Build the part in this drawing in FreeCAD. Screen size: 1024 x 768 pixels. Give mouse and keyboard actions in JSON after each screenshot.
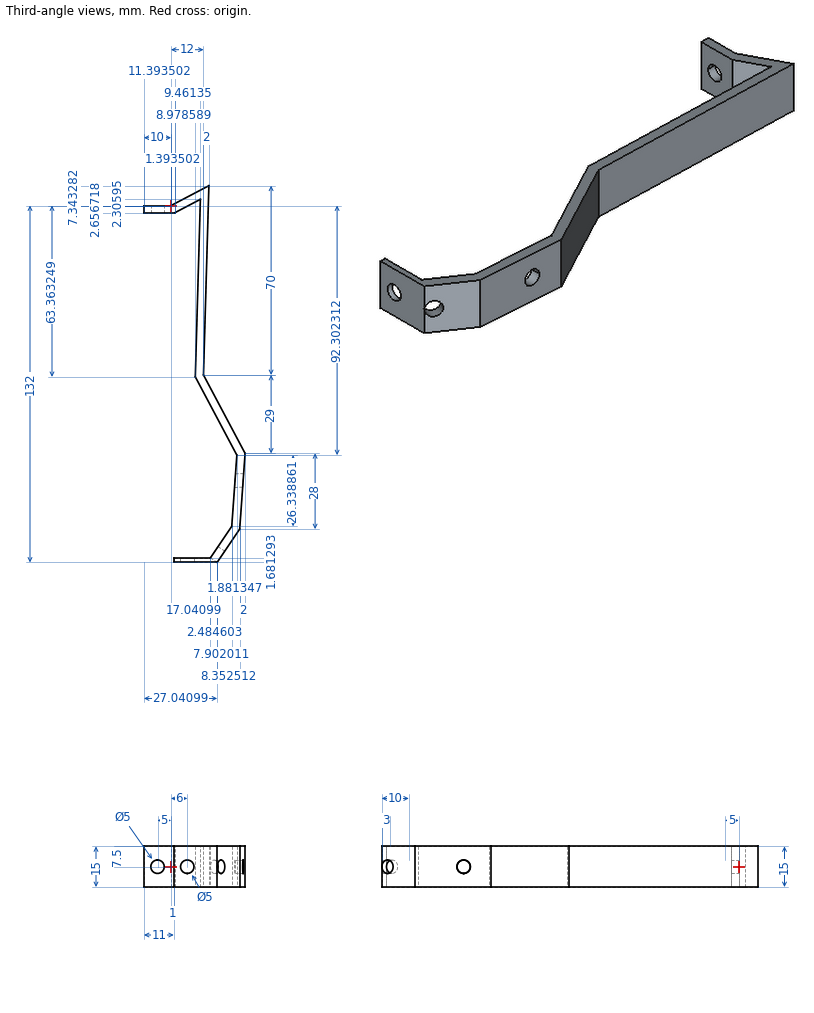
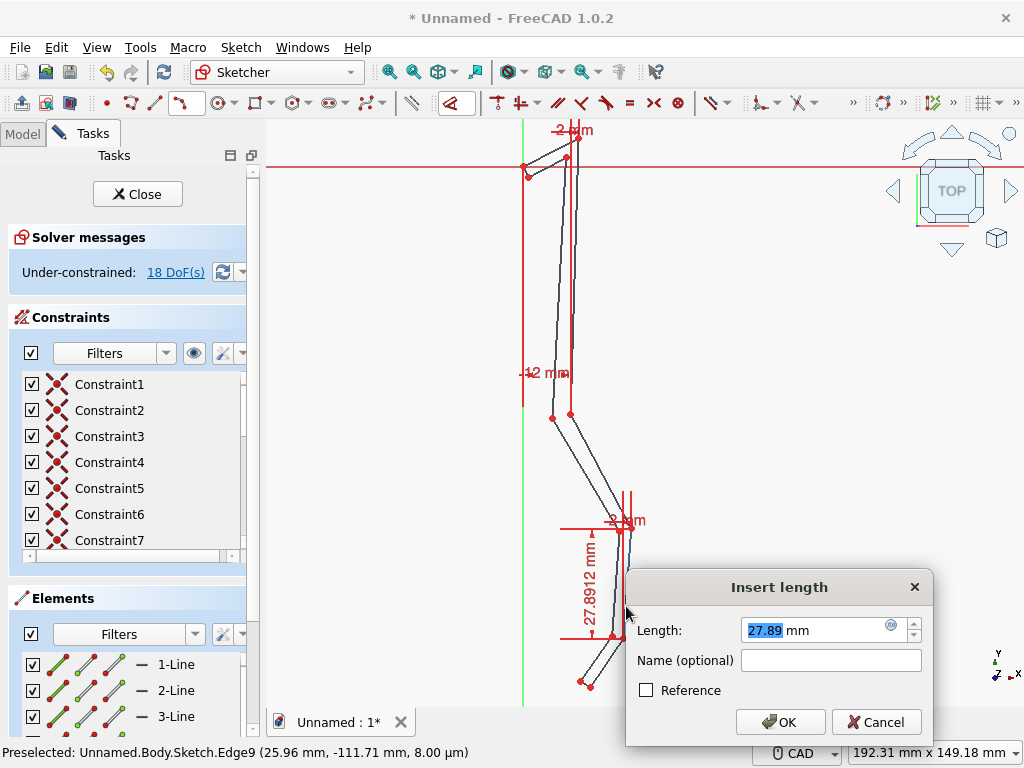
{"action": "type", "text": "28"}
{"action": "key", "text": "Return"}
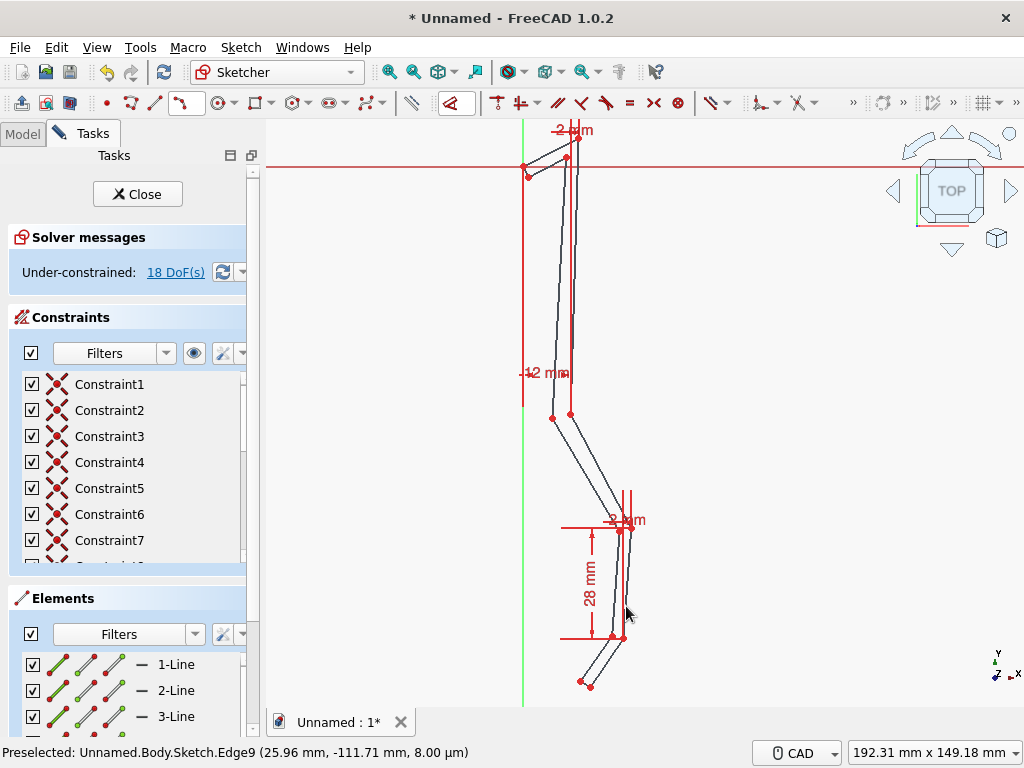
{"action": "left_click", "coordinate": [613, 494]}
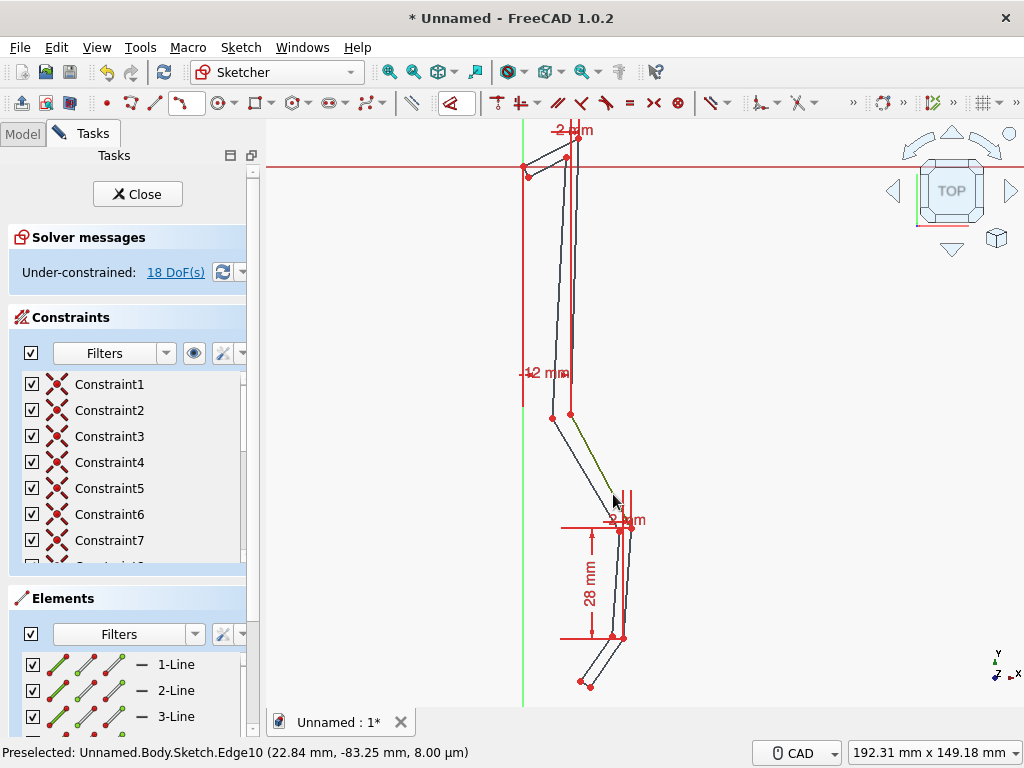
{"action": "key", "text": "i"}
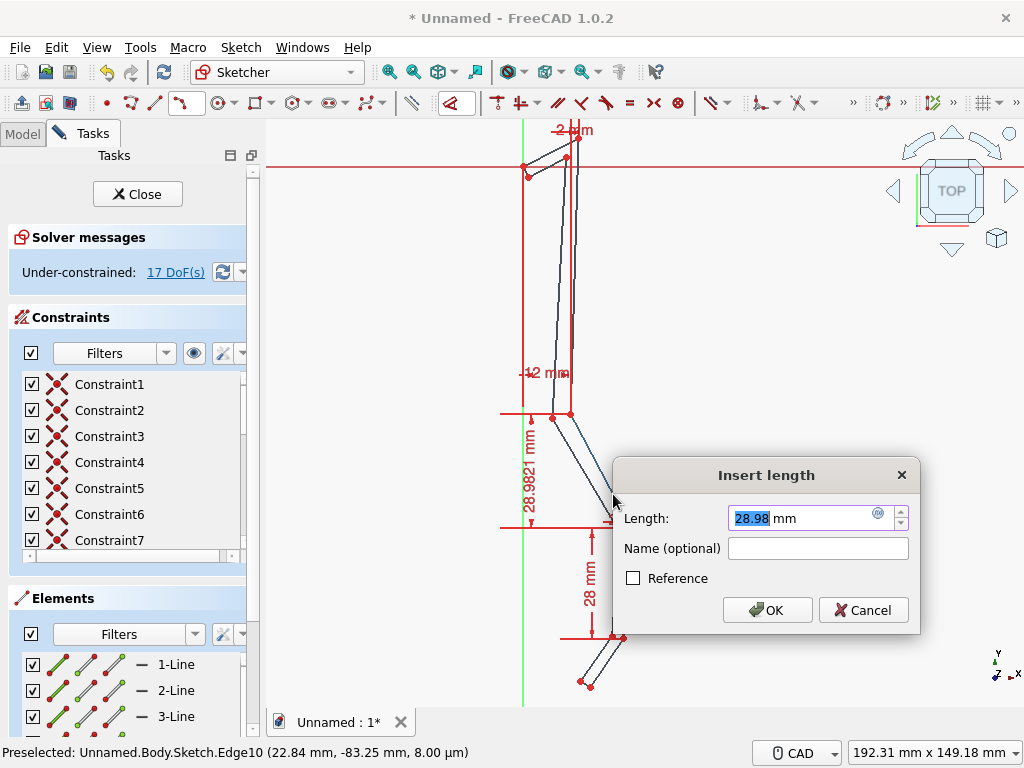
{"action": "type", "text": "29"}
{"action": "key", "text": "Return"}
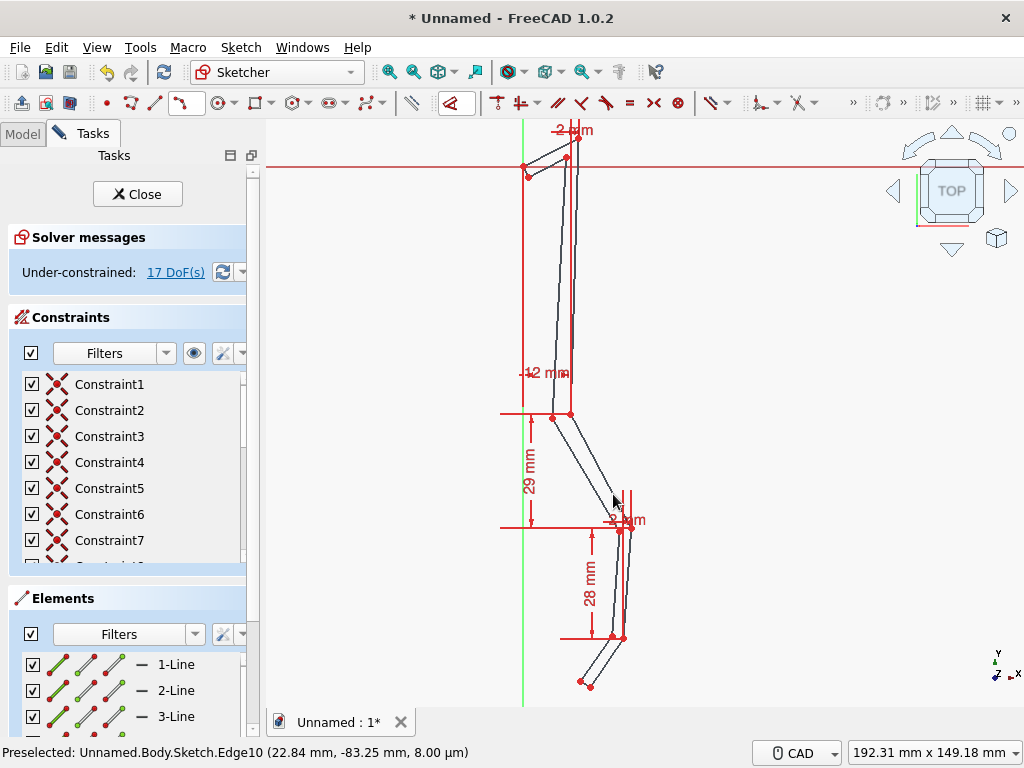
{"action": "left_click", "coordinate": [573, 332]}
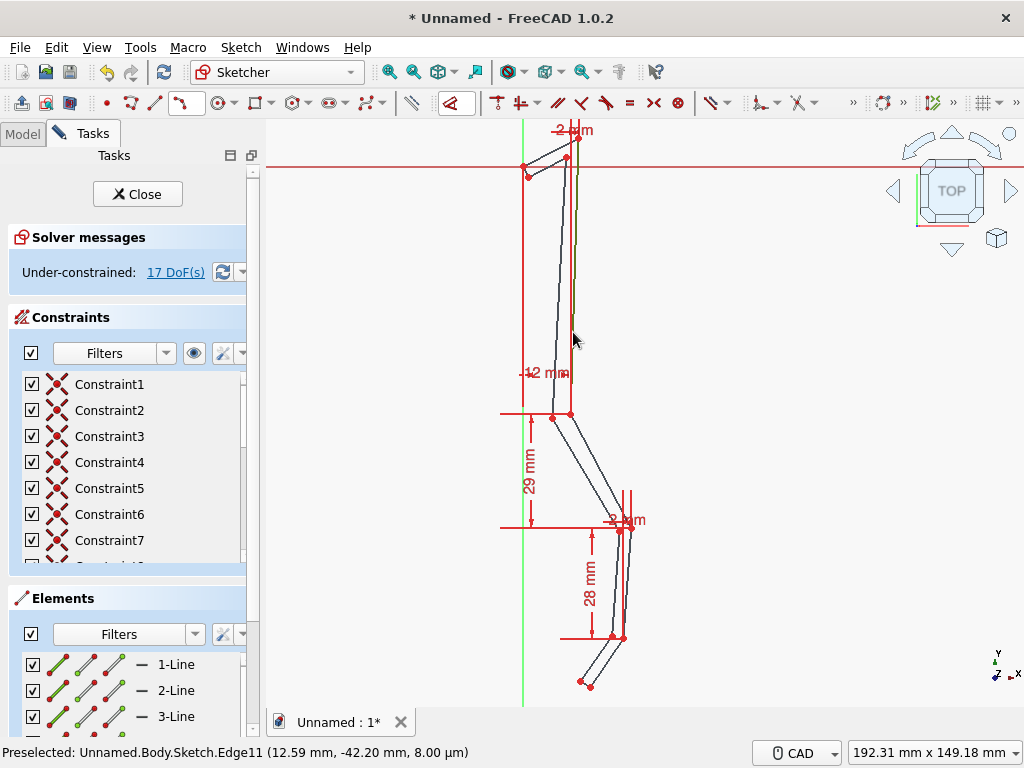
{"action": "left_click", "coordinate": [470, 104]}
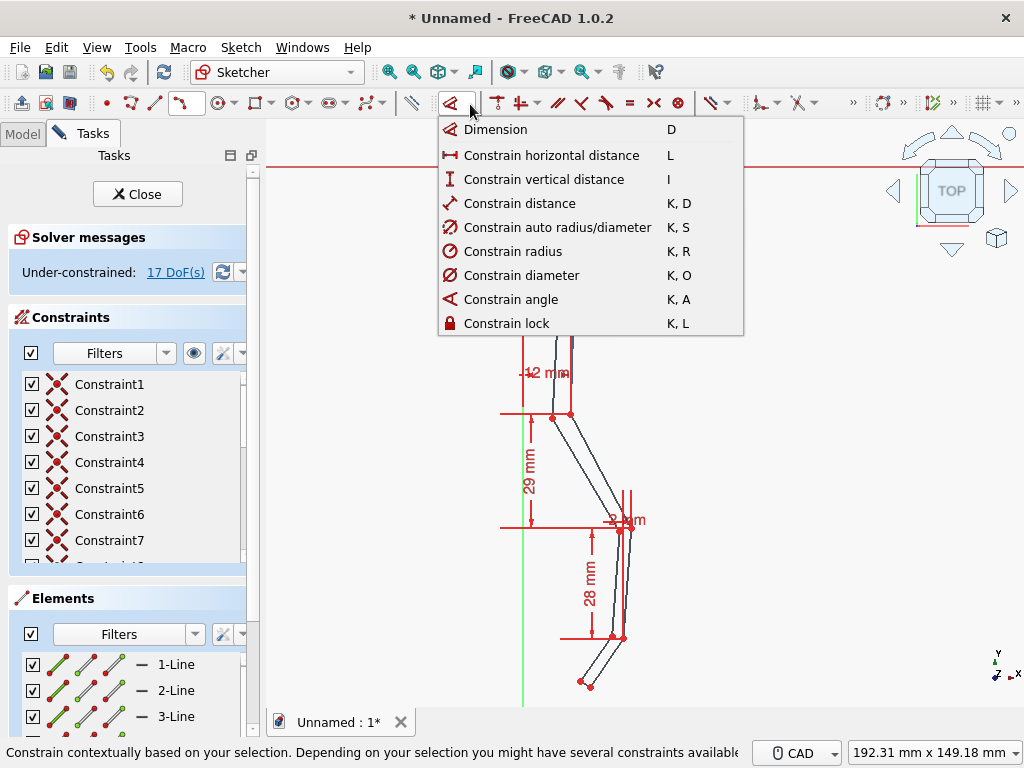
{"action": "left_click", "coordinate": [591, 179]}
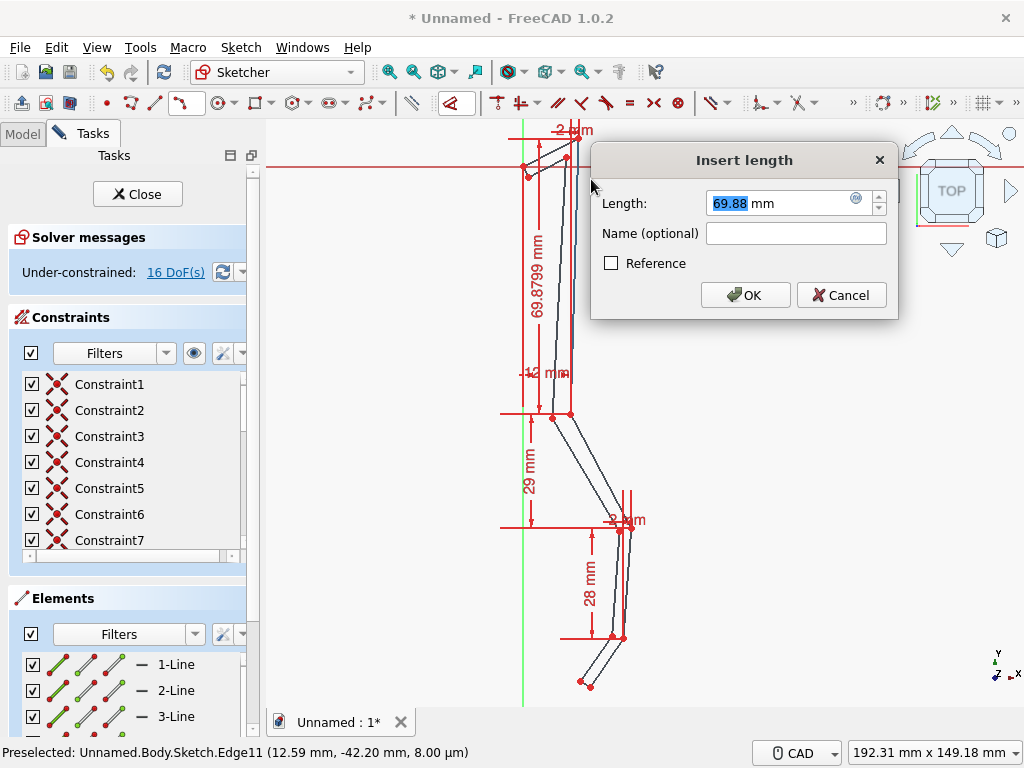
{"action": "type", "text": "70"}
{"action": "key", "text": "Return"}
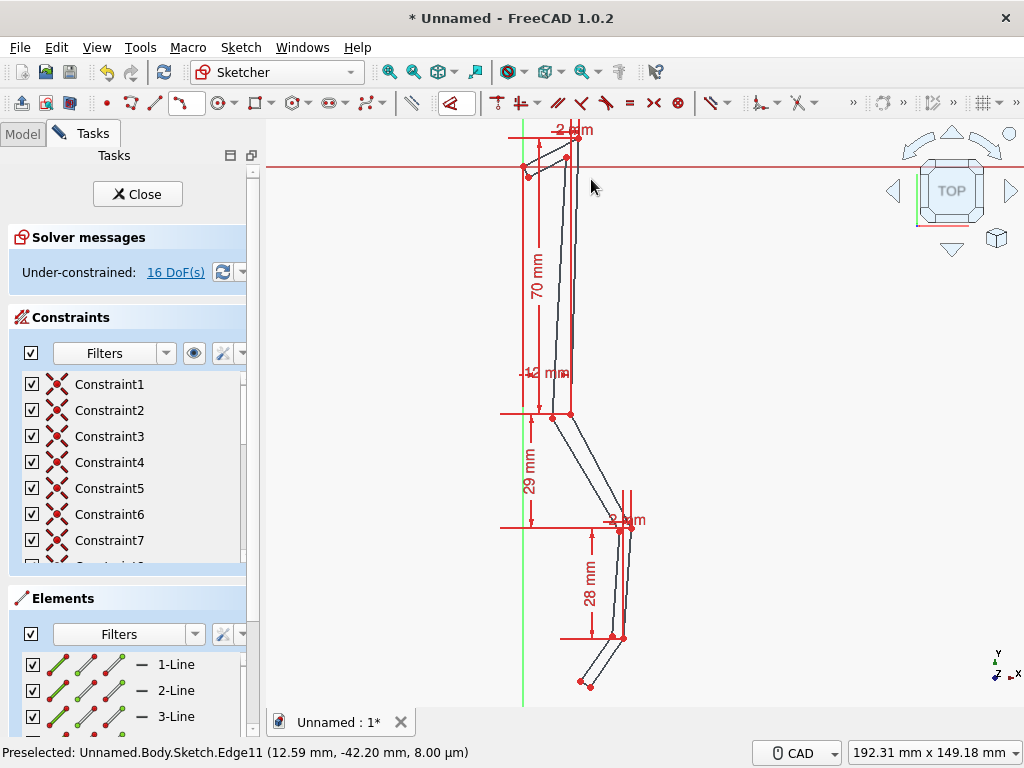
{"action": "scroll", "coordinate": [575, 414], "scroll_direction": "down", "scroll_amount": 2}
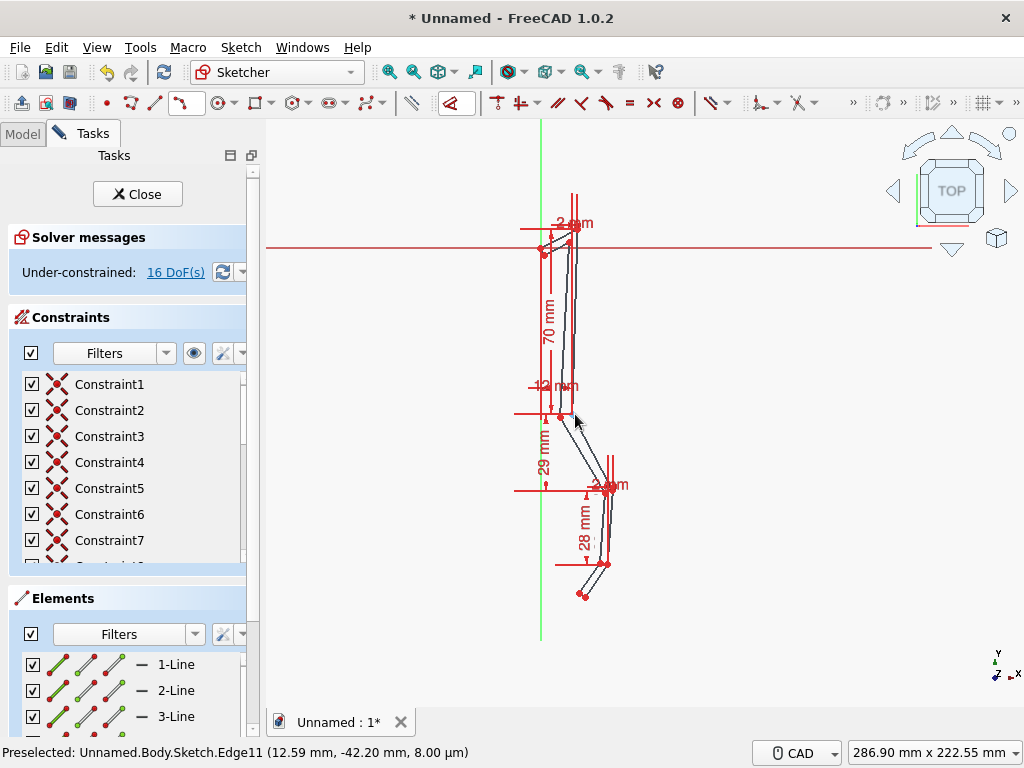
{"action": "scroll", "coordinate": [585, 598], "scroll_direction": "up", "scroll_amount": 3}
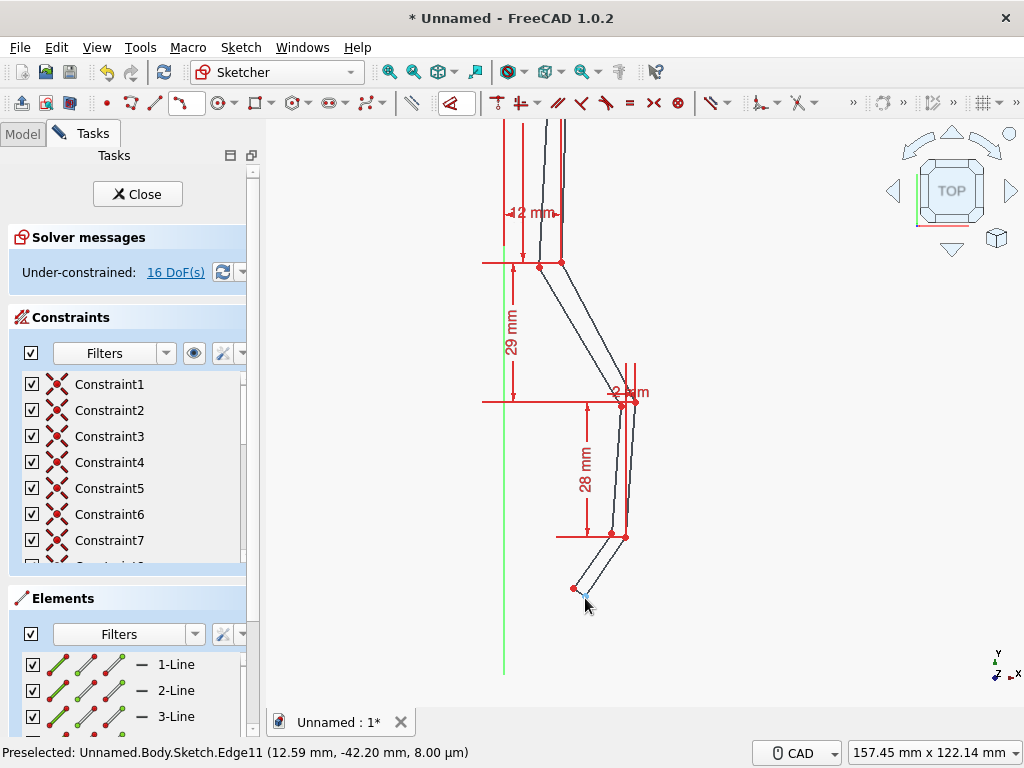
{"action": "left_click", "coordinate": [585, 597]}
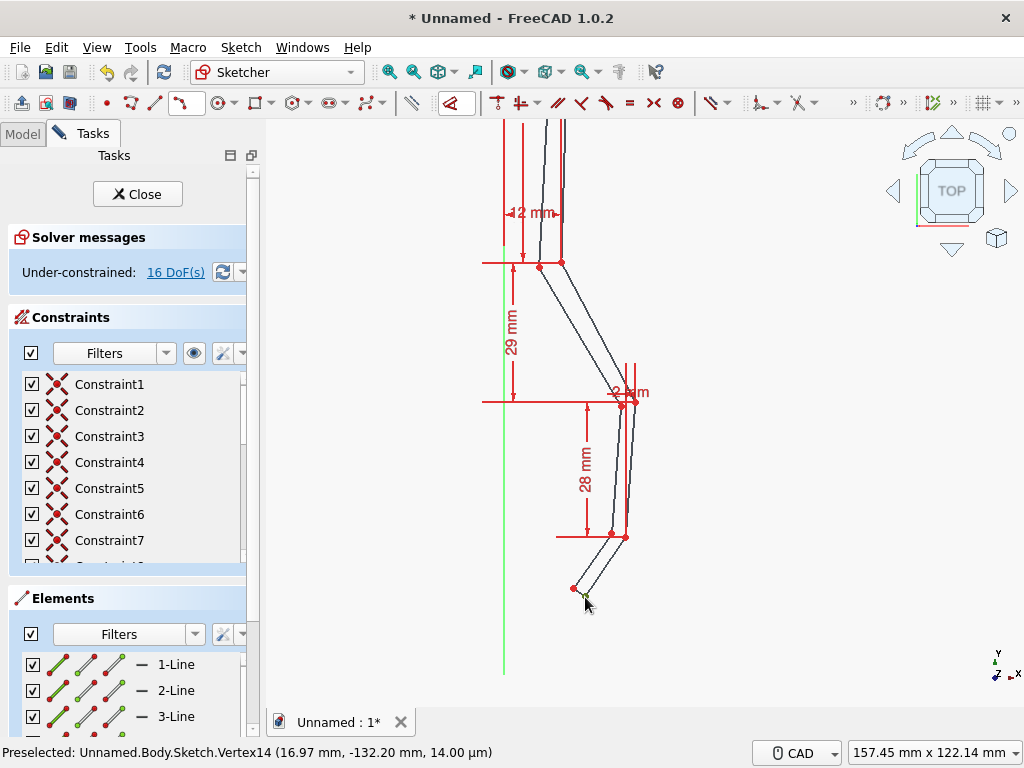
{"action": "left_click", "coordinate": [470, 104]}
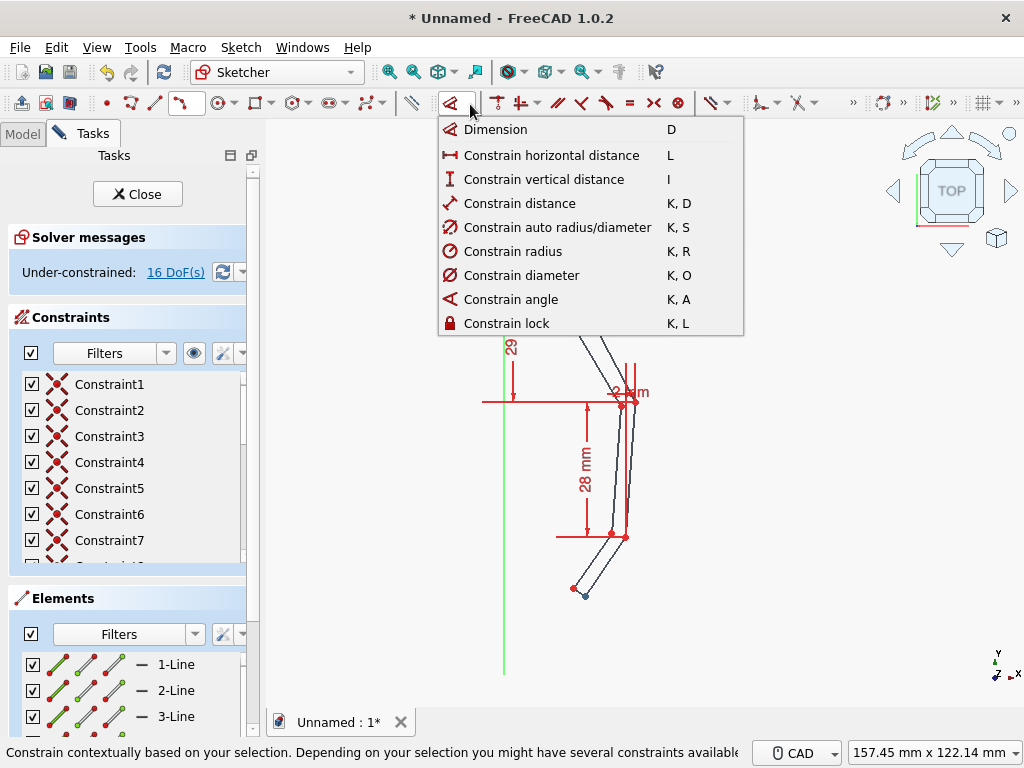
{"action": "left_click", "coordinate": [591, 179]}